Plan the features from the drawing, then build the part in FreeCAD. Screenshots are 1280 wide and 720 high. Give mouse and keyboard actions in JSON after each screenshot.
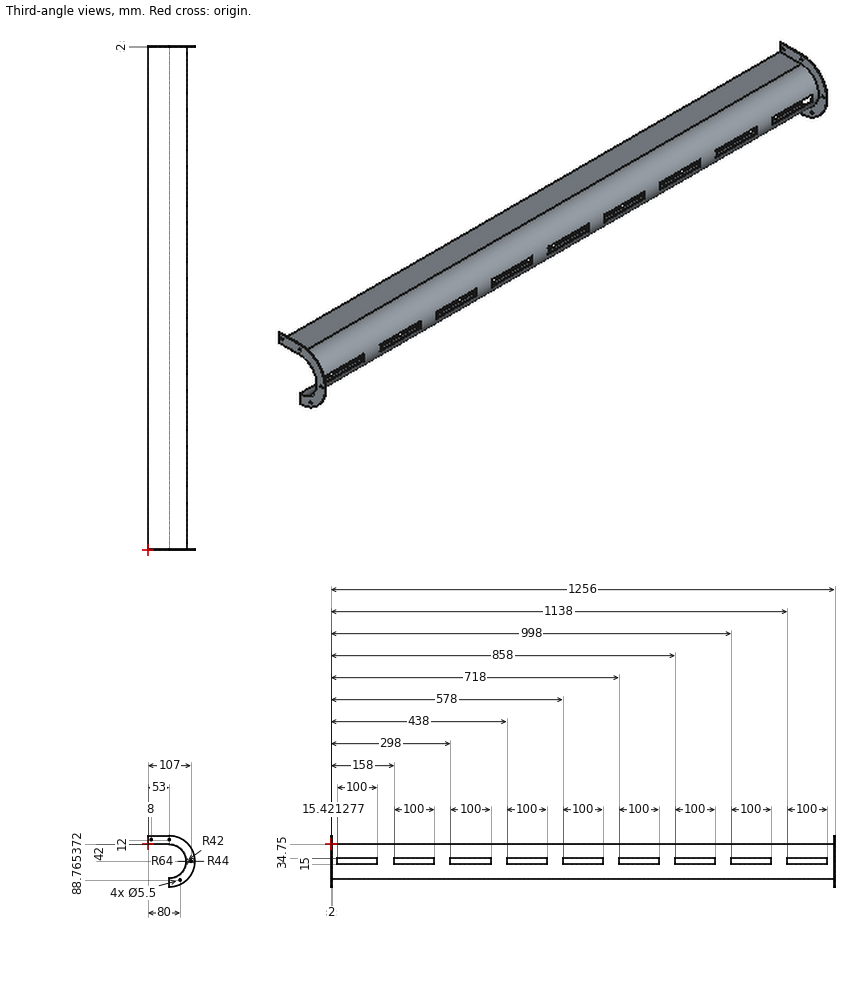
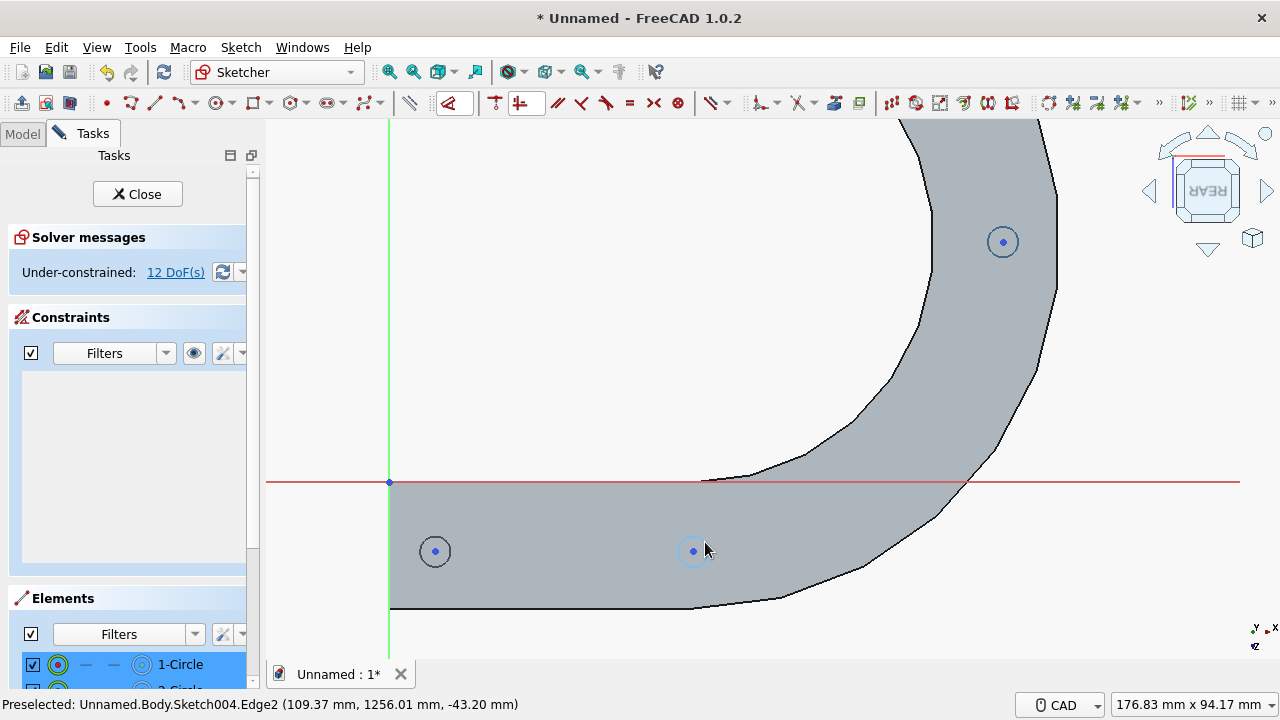
{"action": "left_click", "coordinate": [704, 541]}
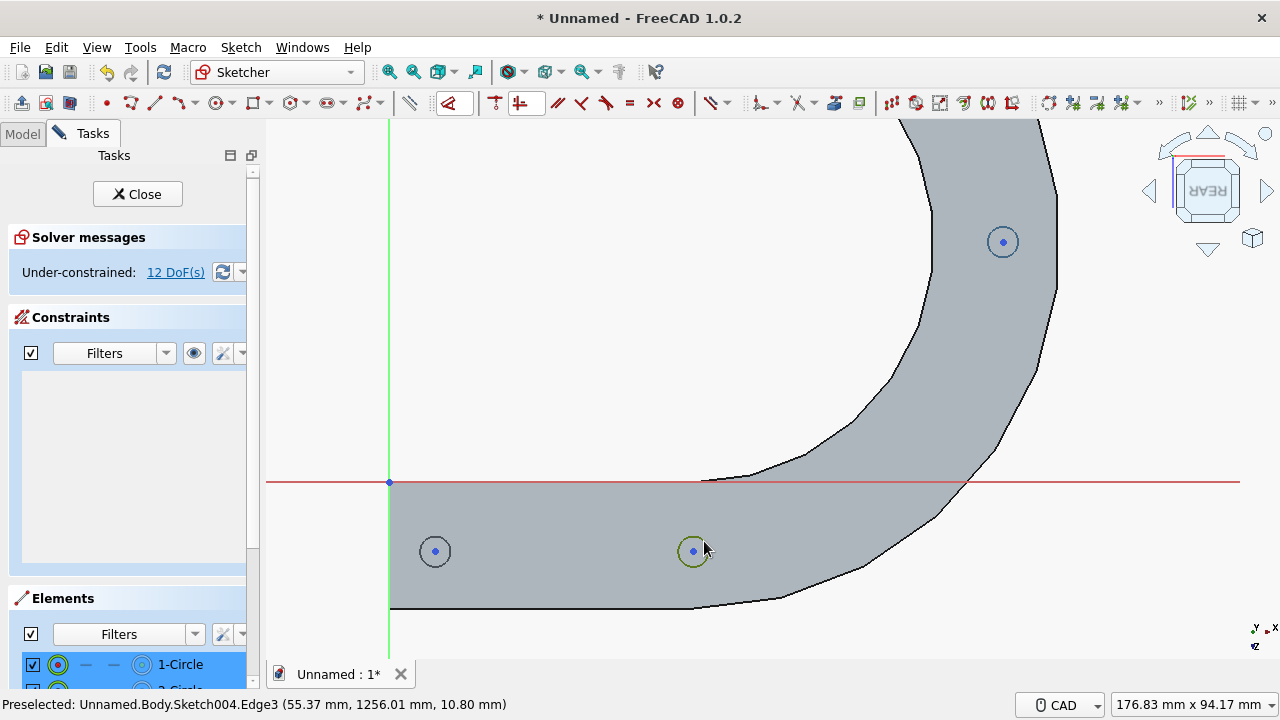
{"action": "left_click", "coordinate": [446, 541]}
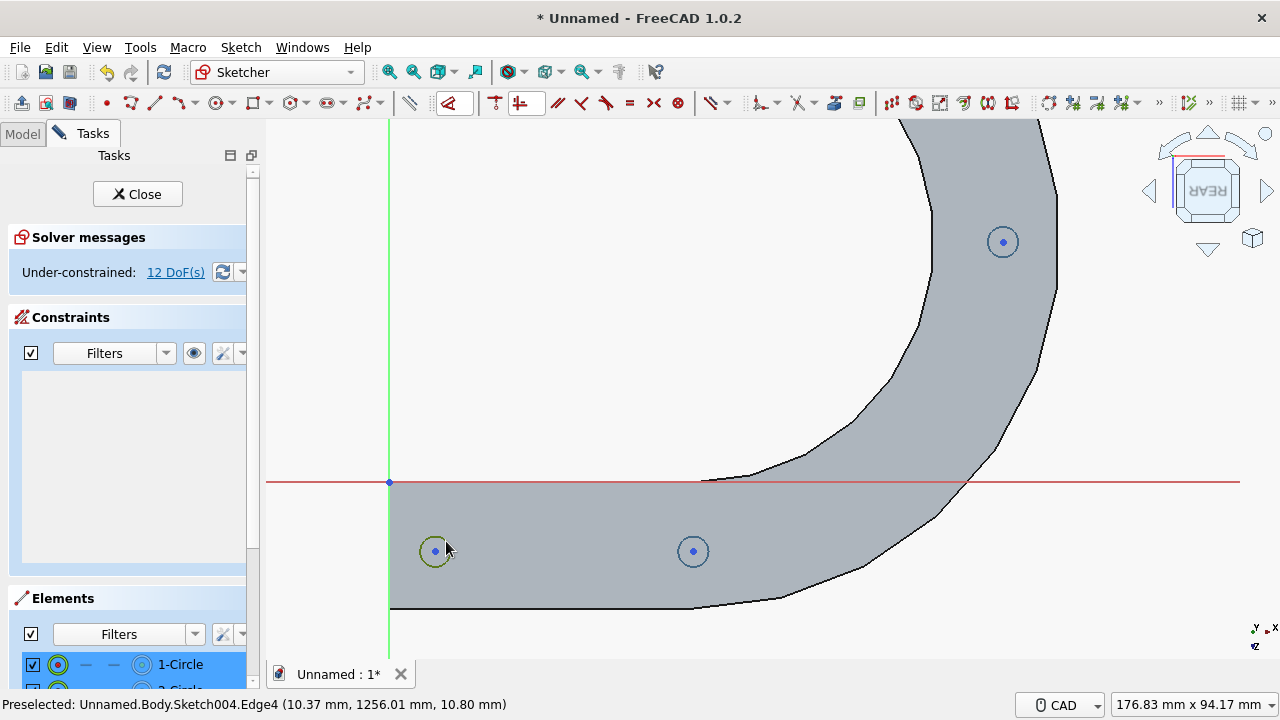
{"action": "left_click", "coordinate": [630, 104]}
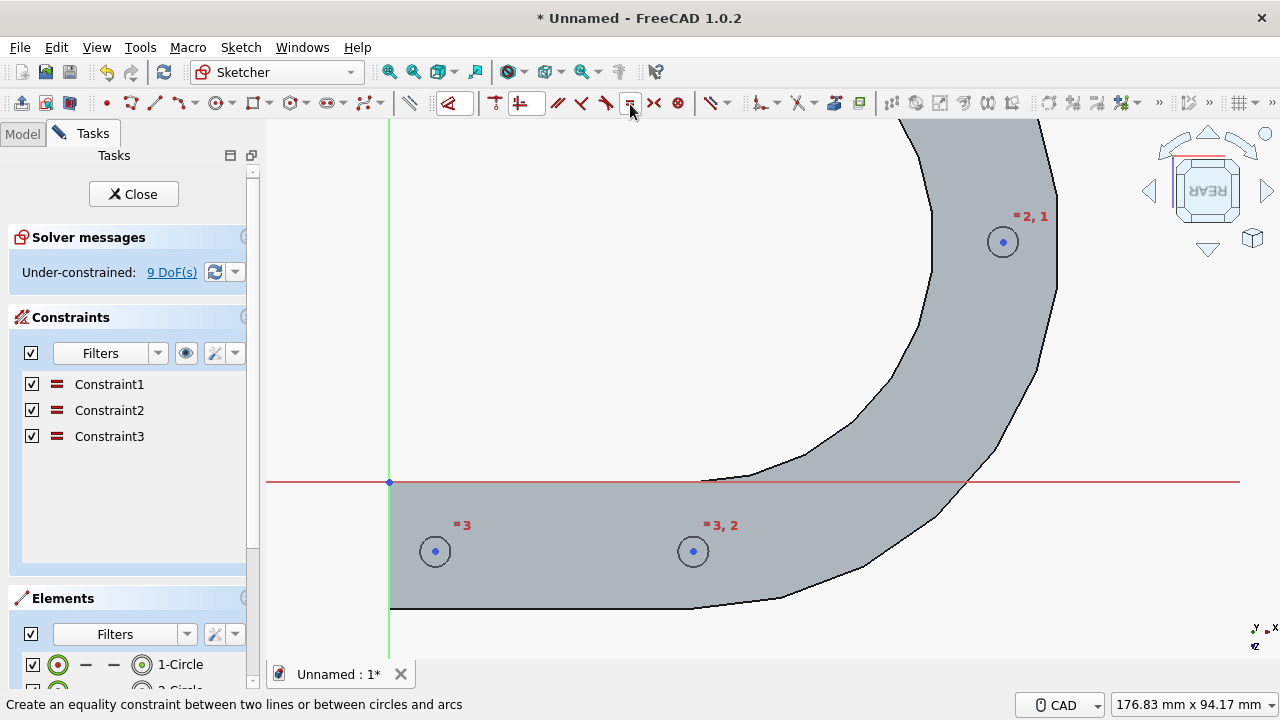
{"action": "left_click", "coordinate": [693, 552]}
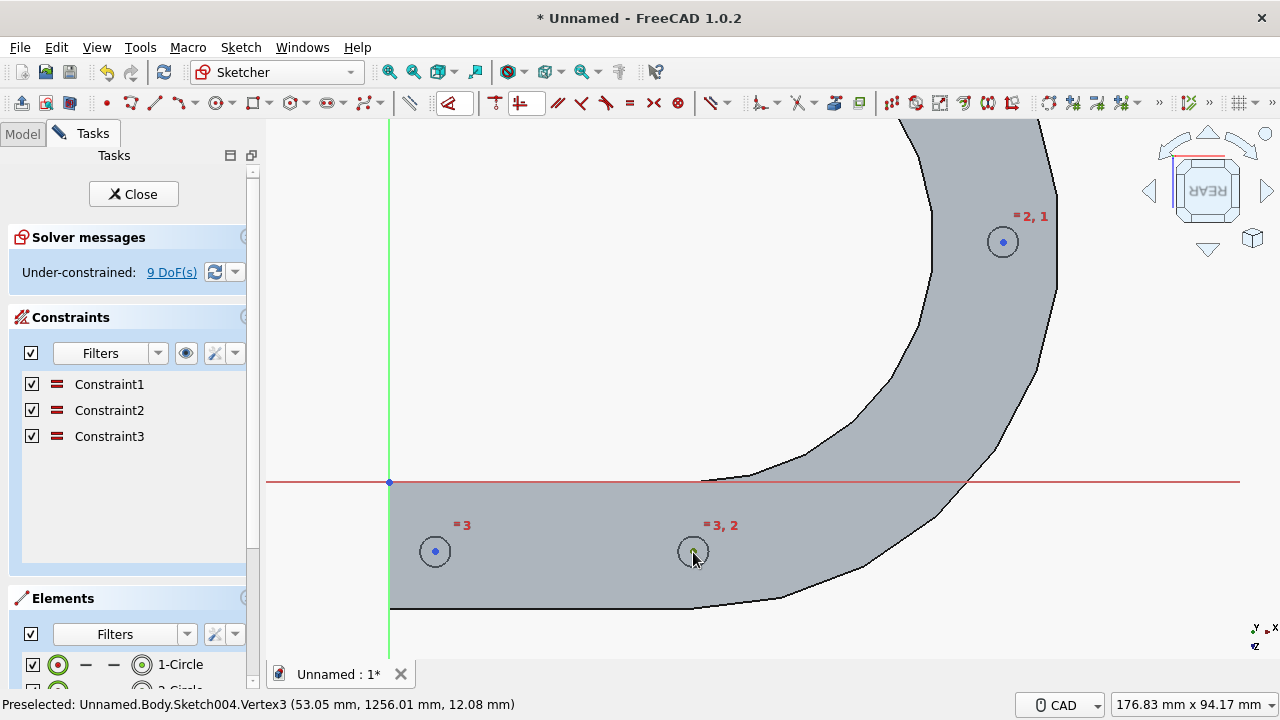
{"action": "left_click", "coordinate": [435, 552]}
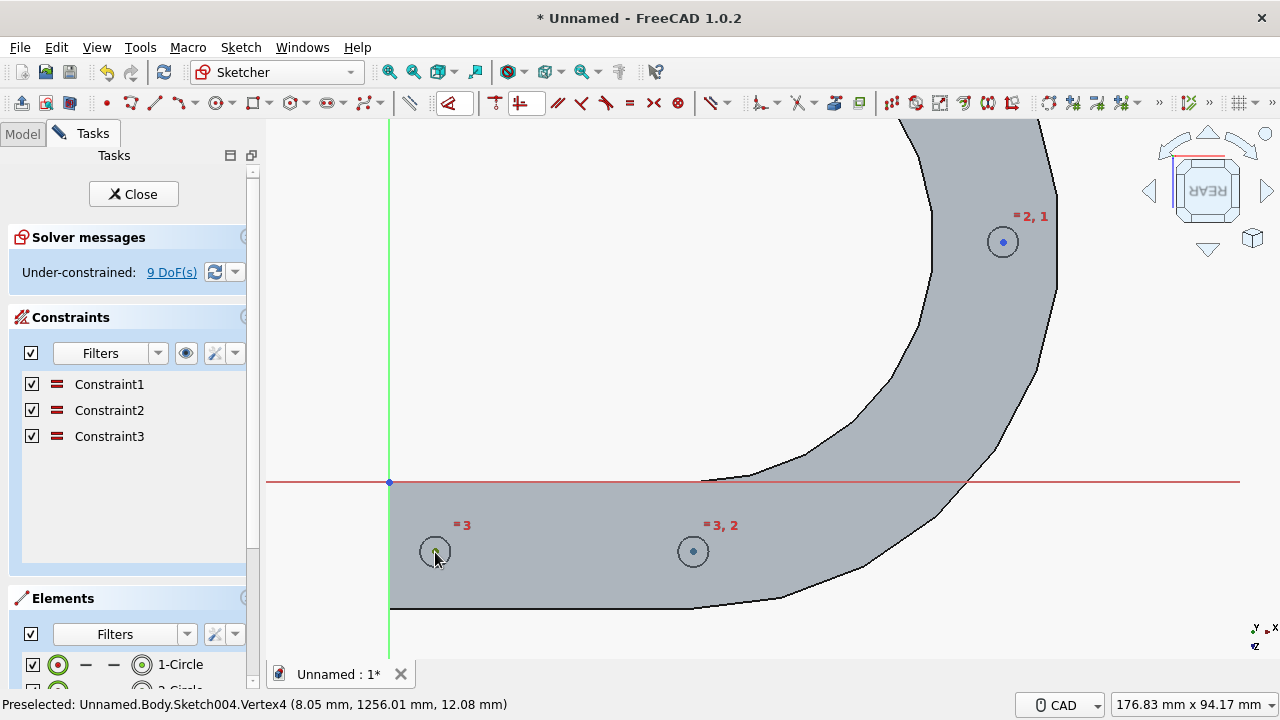
{"action": "key", "text": "h"}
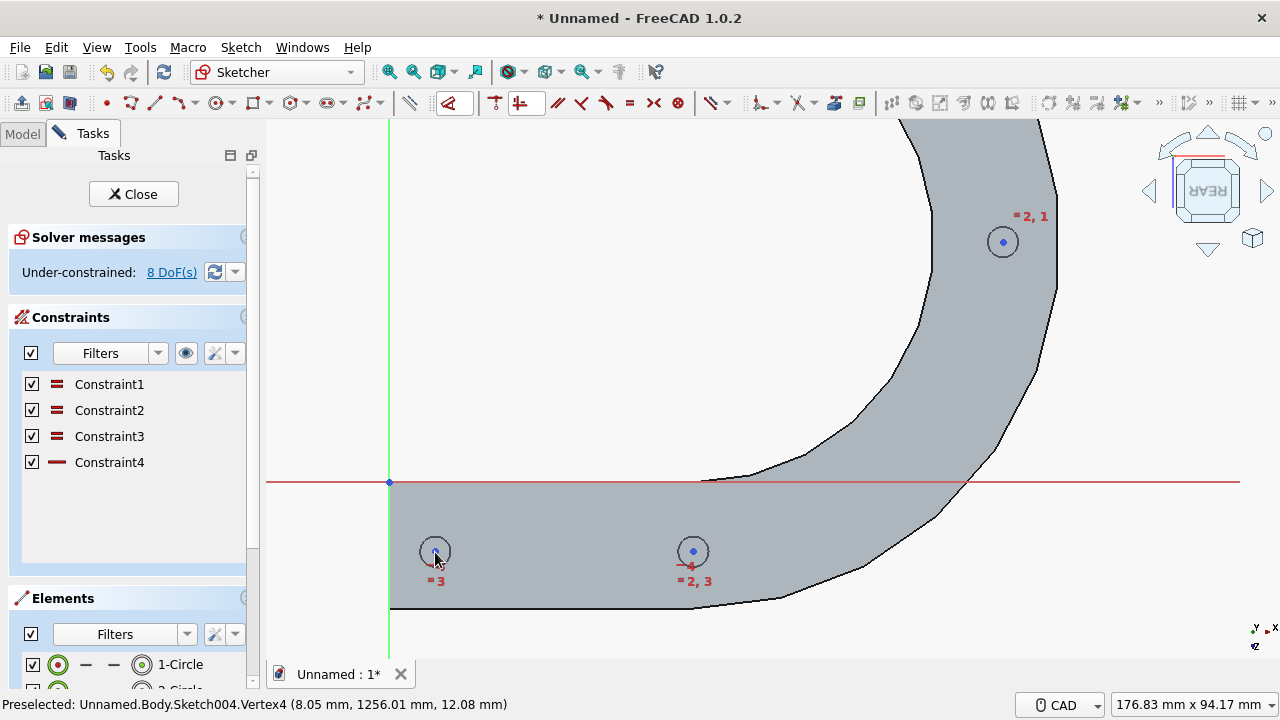
{"action": "scroll", "coordinate": [705, 543], "scroll_direction": "down", "scroll_amount": 3}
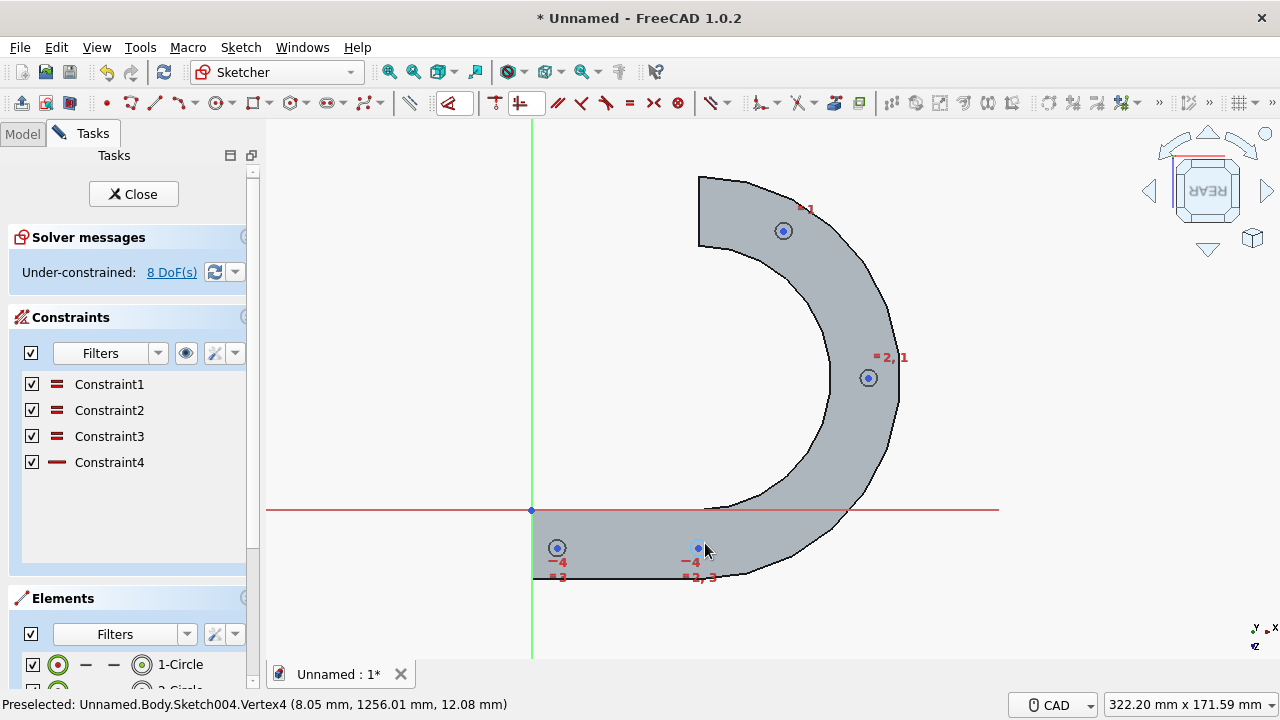
{"action": "scroll", "coordinate": [790, 225], "scroll_direction": "up", "scroll_amount": 5}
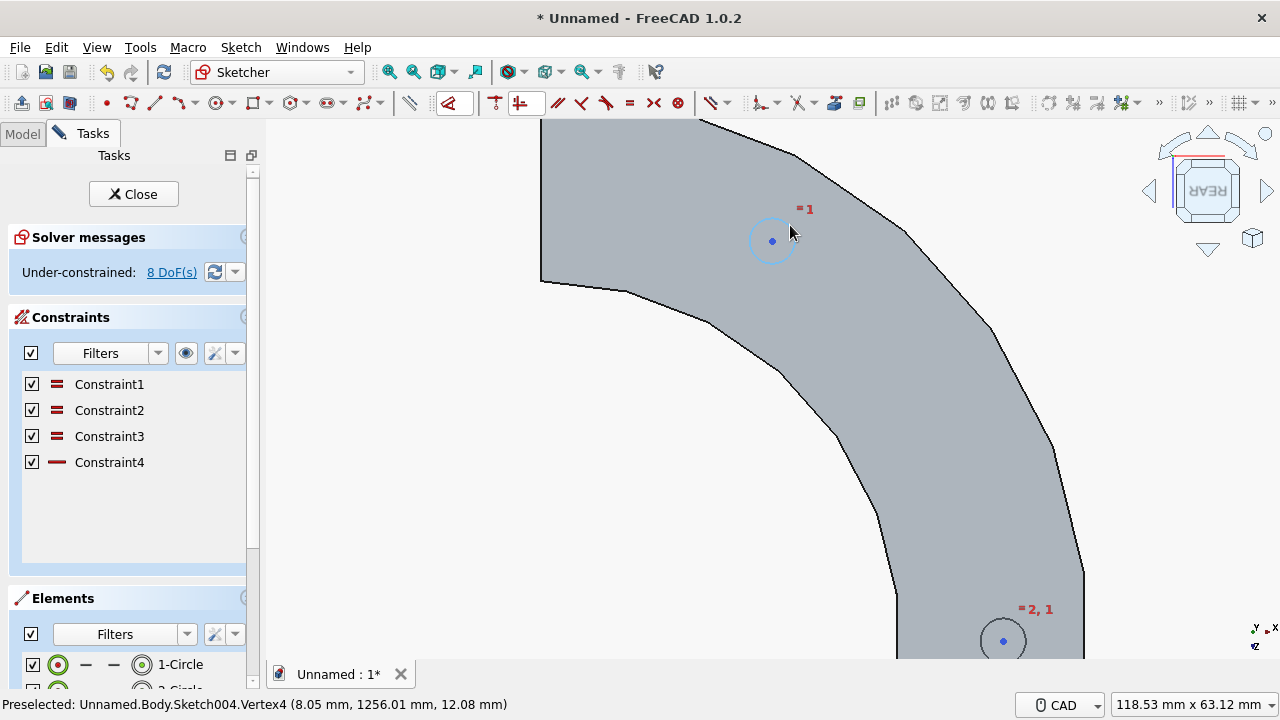
{"action": "left_click", "coordinate": [788, 225]}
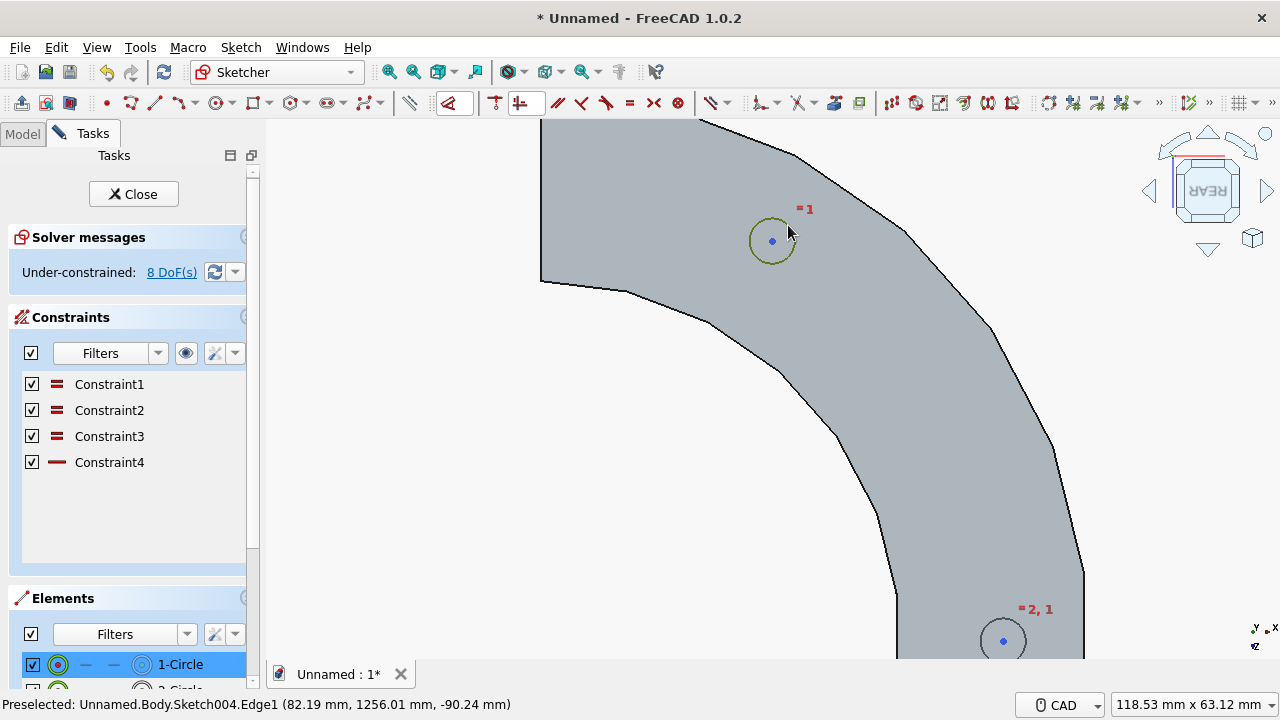
{"action": "key", "text": "k o"}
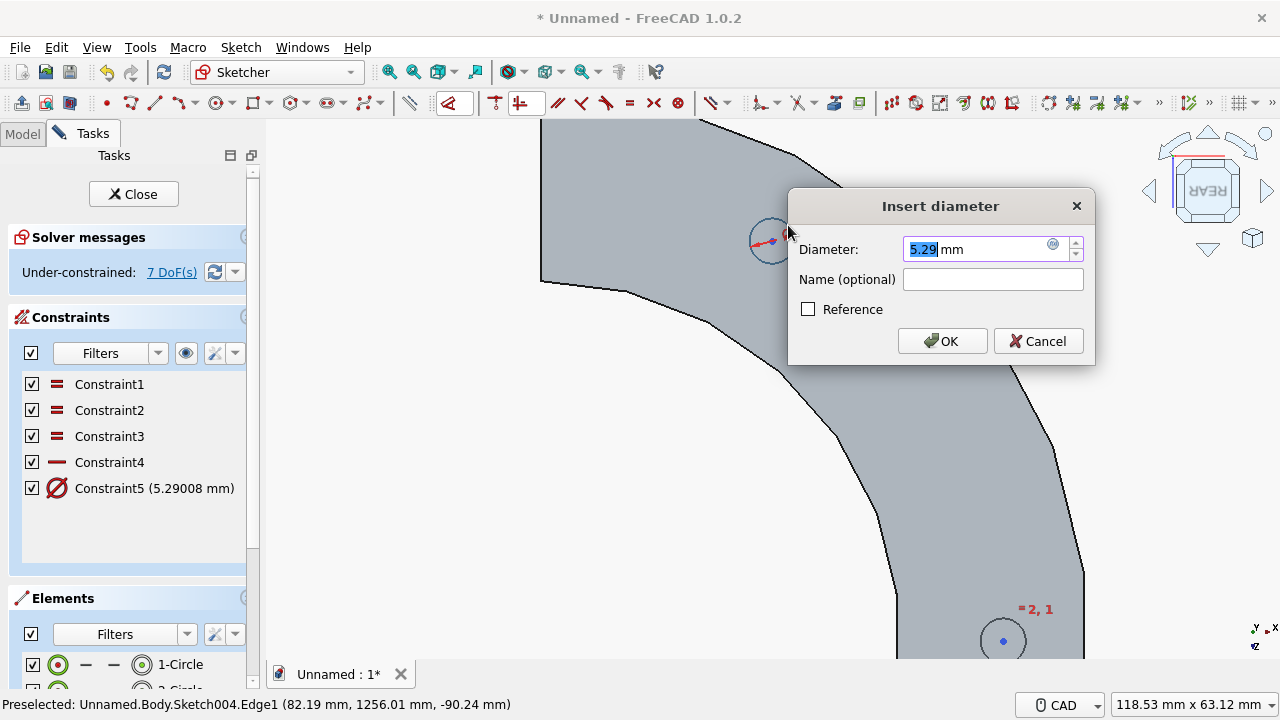
{"action": "type", "text": "5.5"}
{"action": "key", "text": "Return"}